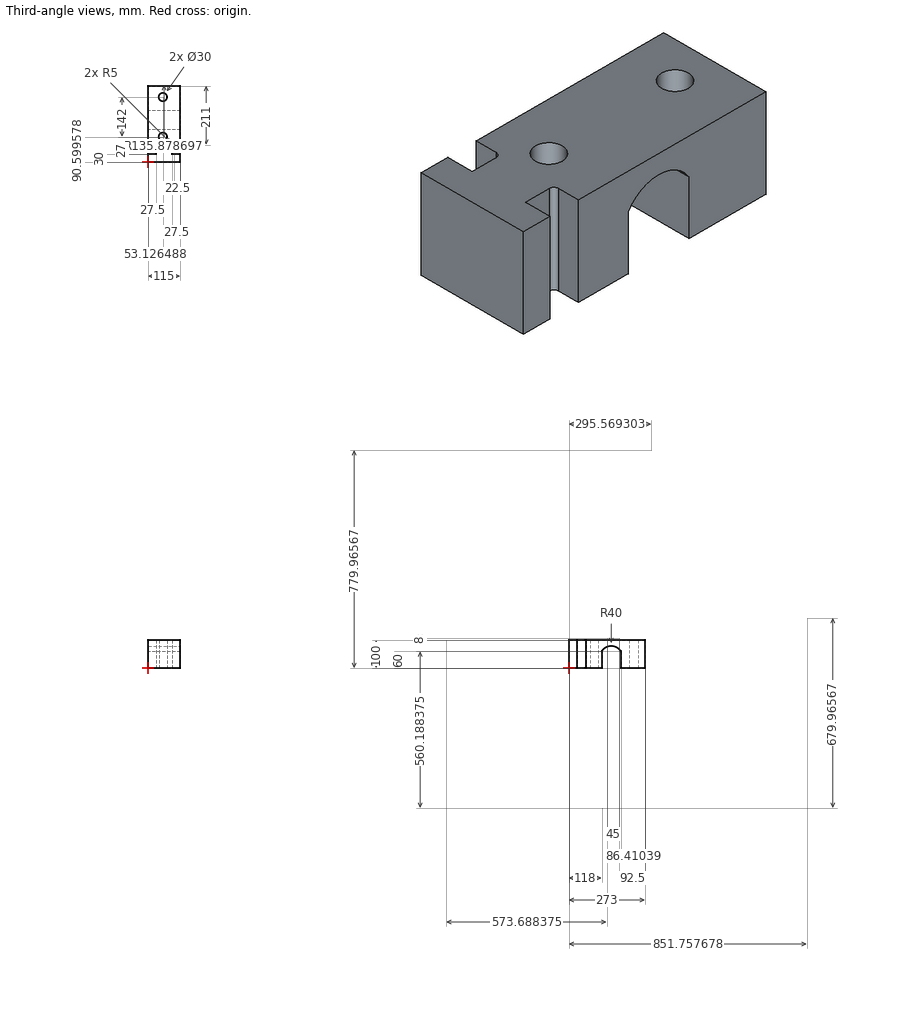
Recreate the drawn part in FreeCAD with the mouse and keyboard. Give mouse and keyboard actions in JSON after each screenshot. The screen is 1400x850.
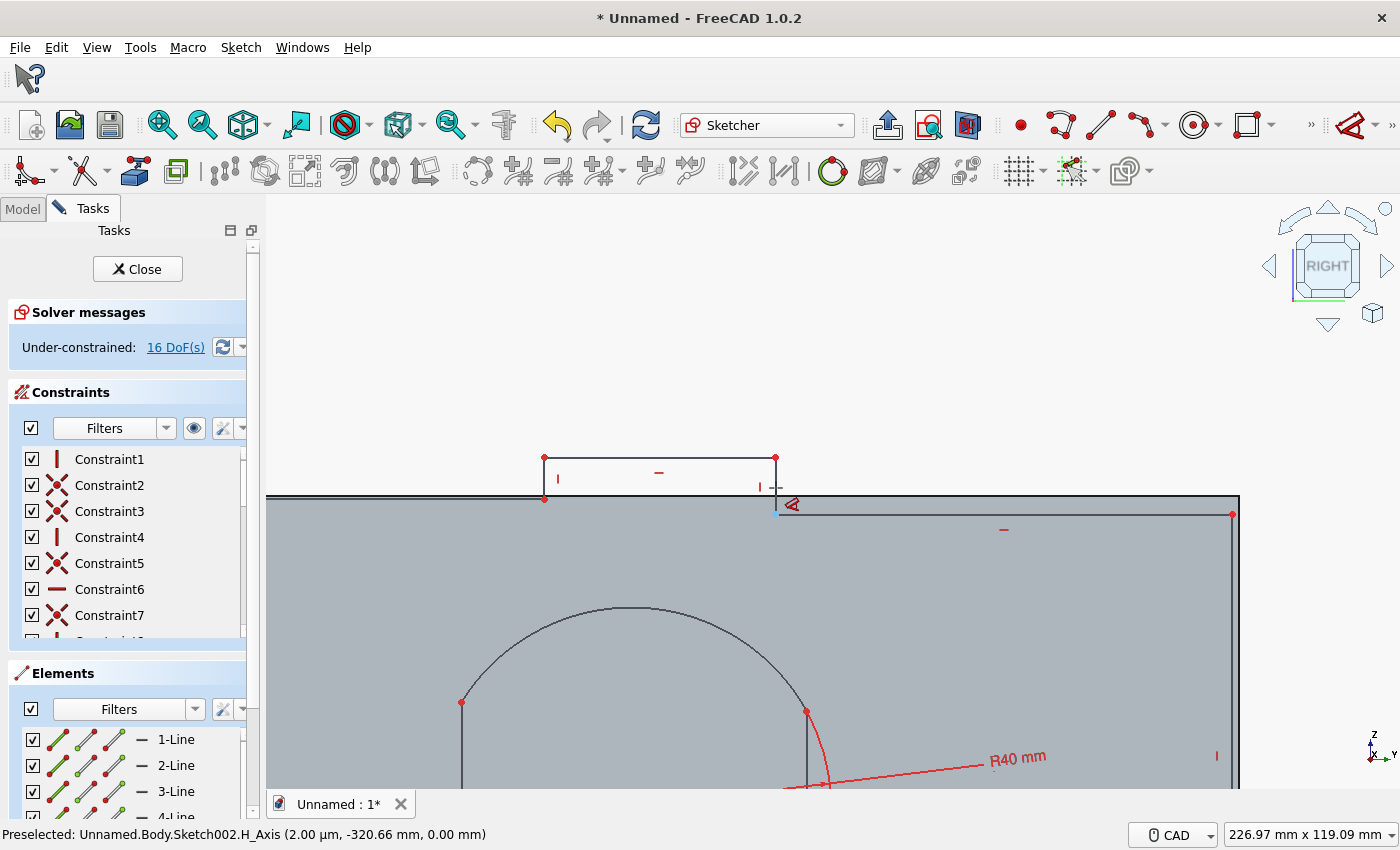
{"action": "left_click", "coordinate": [776, 486]}
{"action": "left_click", "coordinate": [742, 486]}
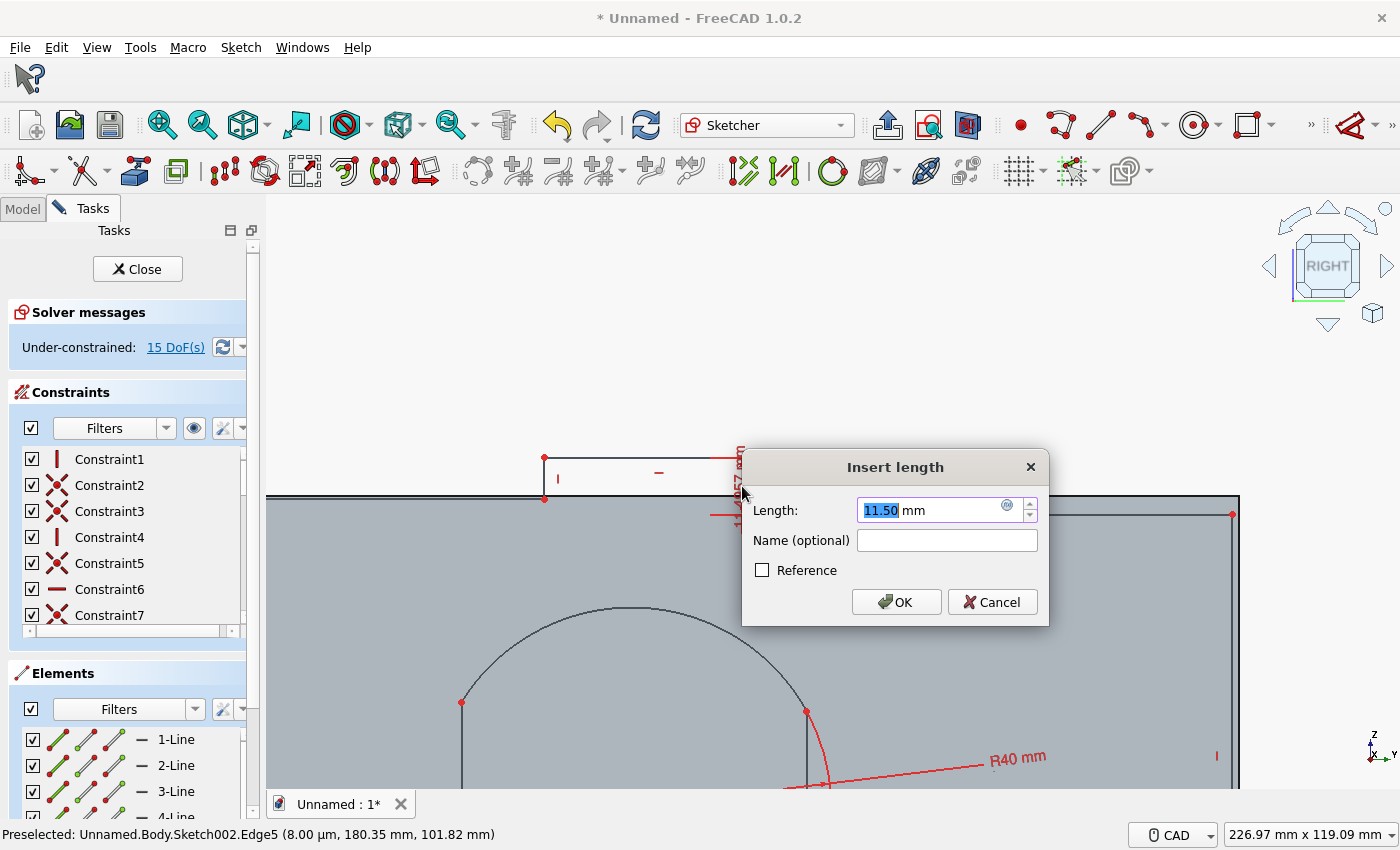
{"action": "type", "text": "8"}
{"action": "key", "text": "Return"}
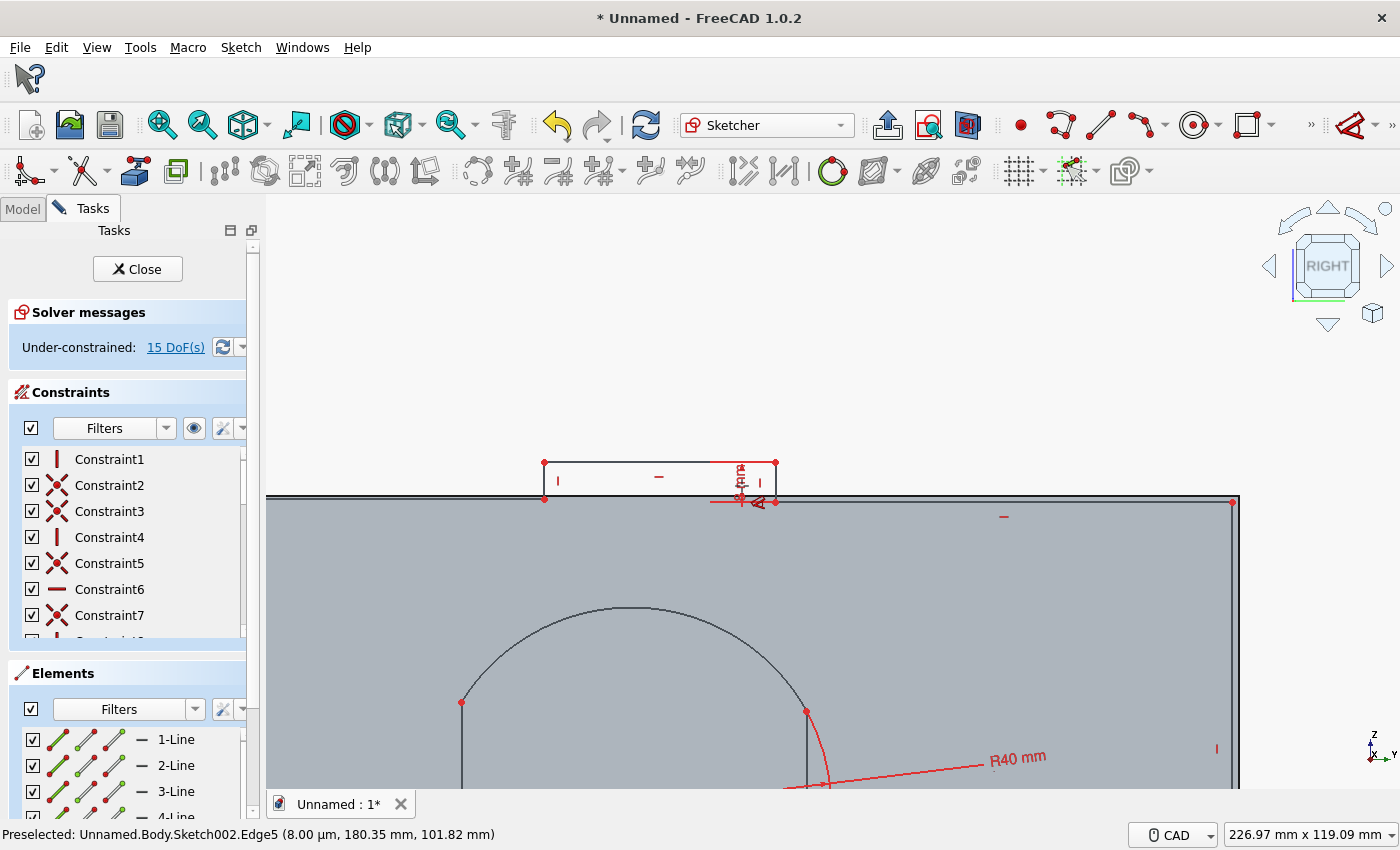
{"action": "left_click", "coordinate": [544, 473]}
{"action": "left_click", "coordinate": [510, 481]}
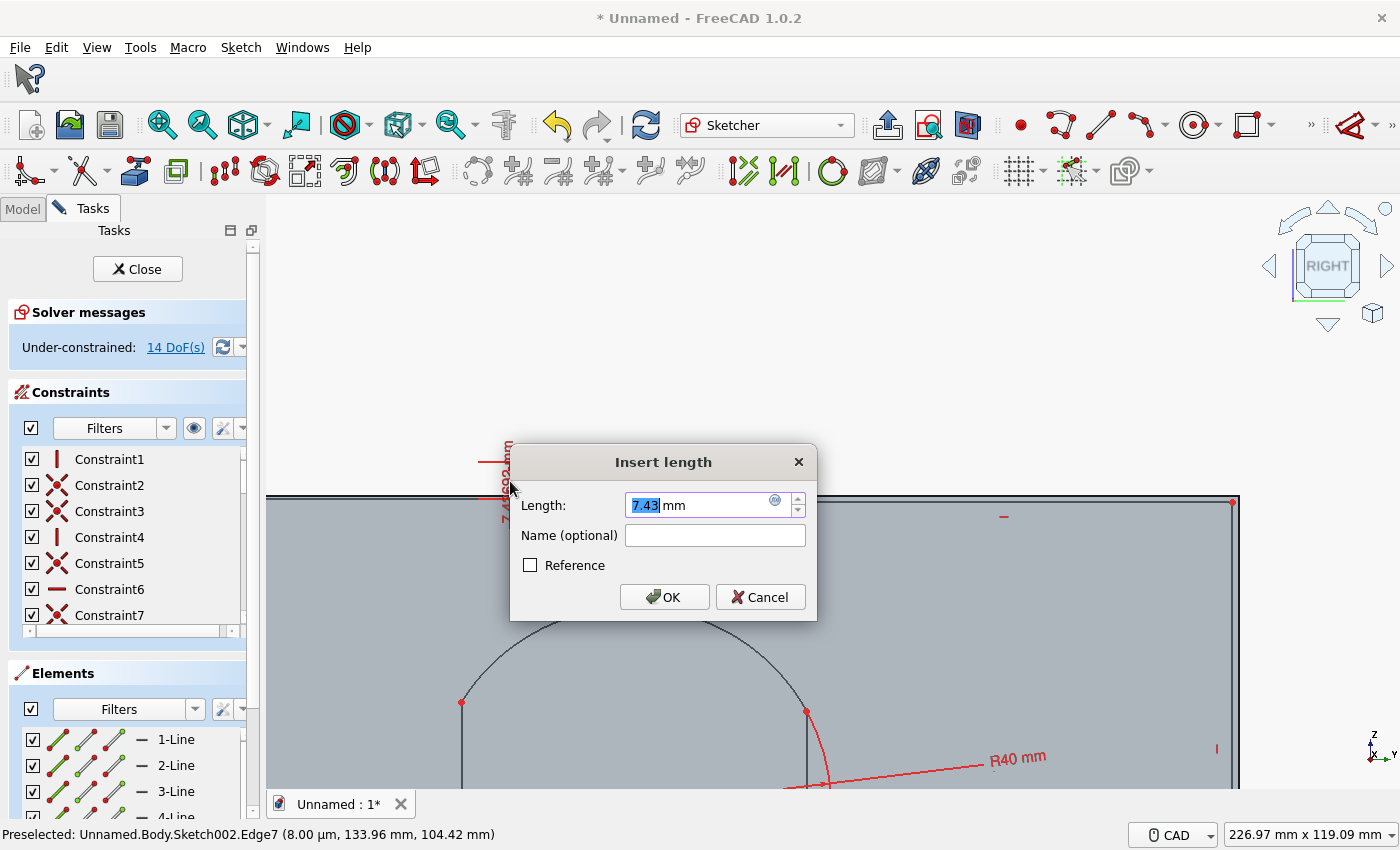
{"action": "type", "text": "8"}
{"action": "key", "text": "Return"}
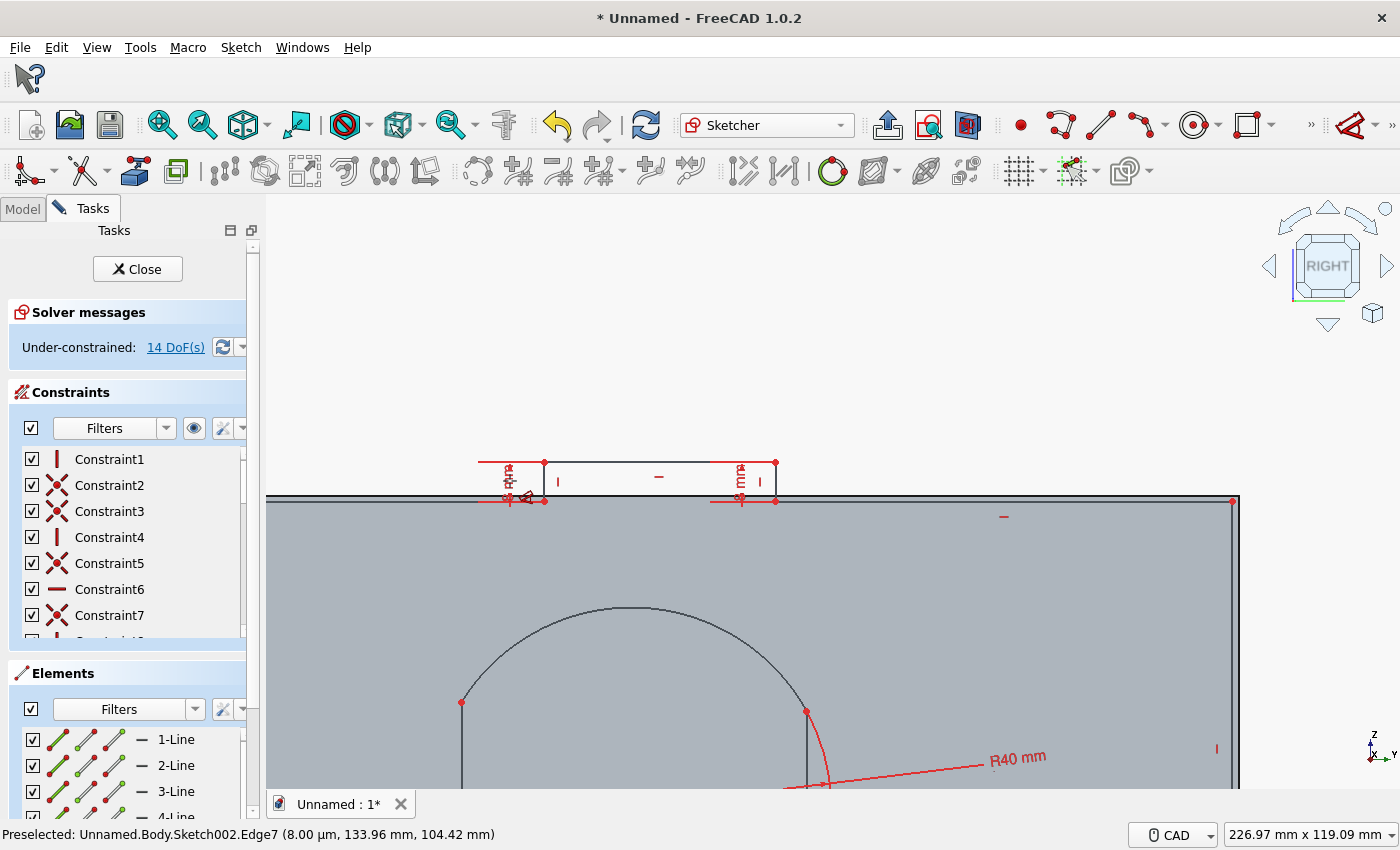
{"action": "scroll", "coordinate": [755, 504], "scroll_direction": "down", "scroll_amount": 14}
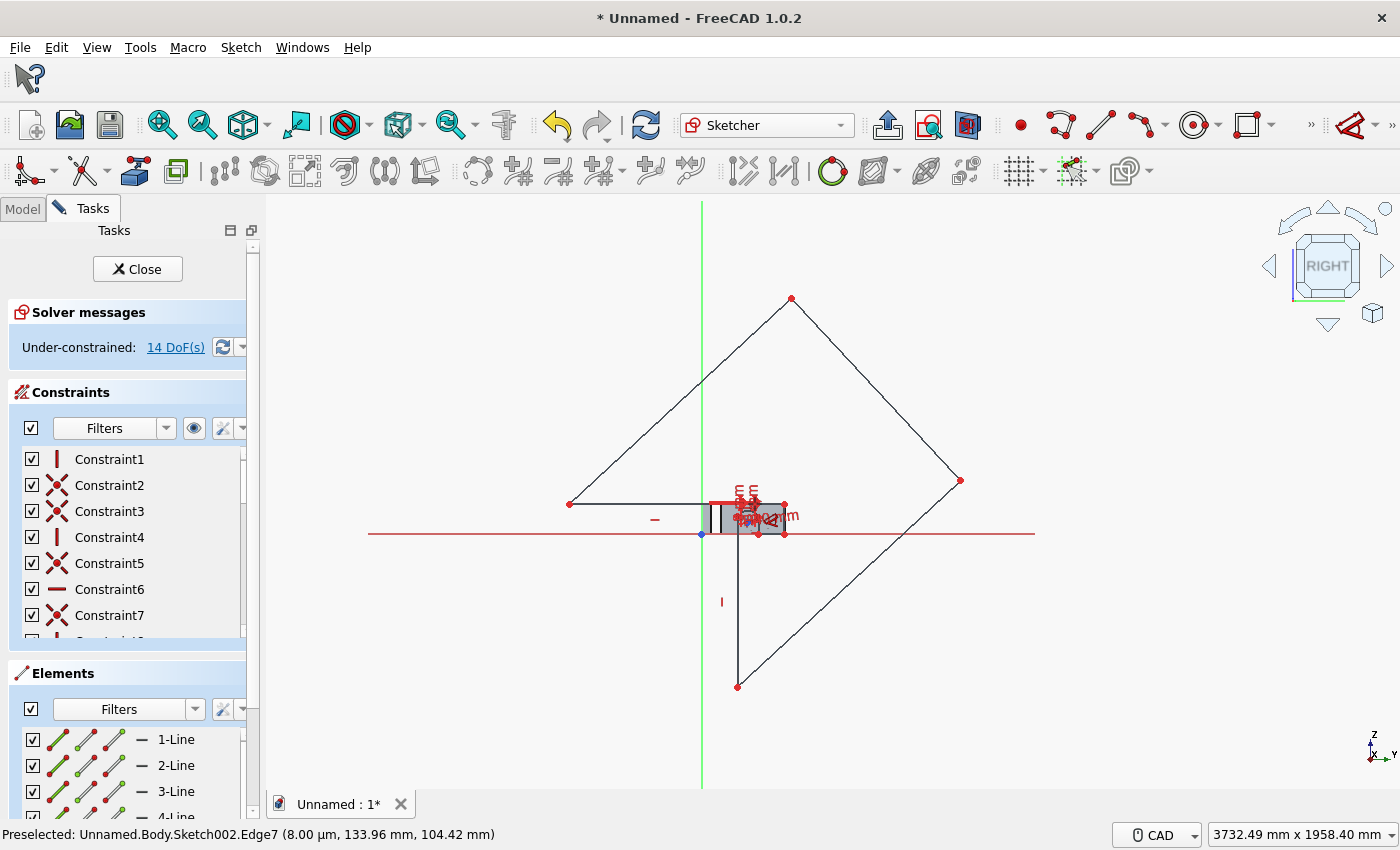
{"action": "scroll", "coordinate": [759, 522], "scroll_direction": "up", "scroll_amount": 5}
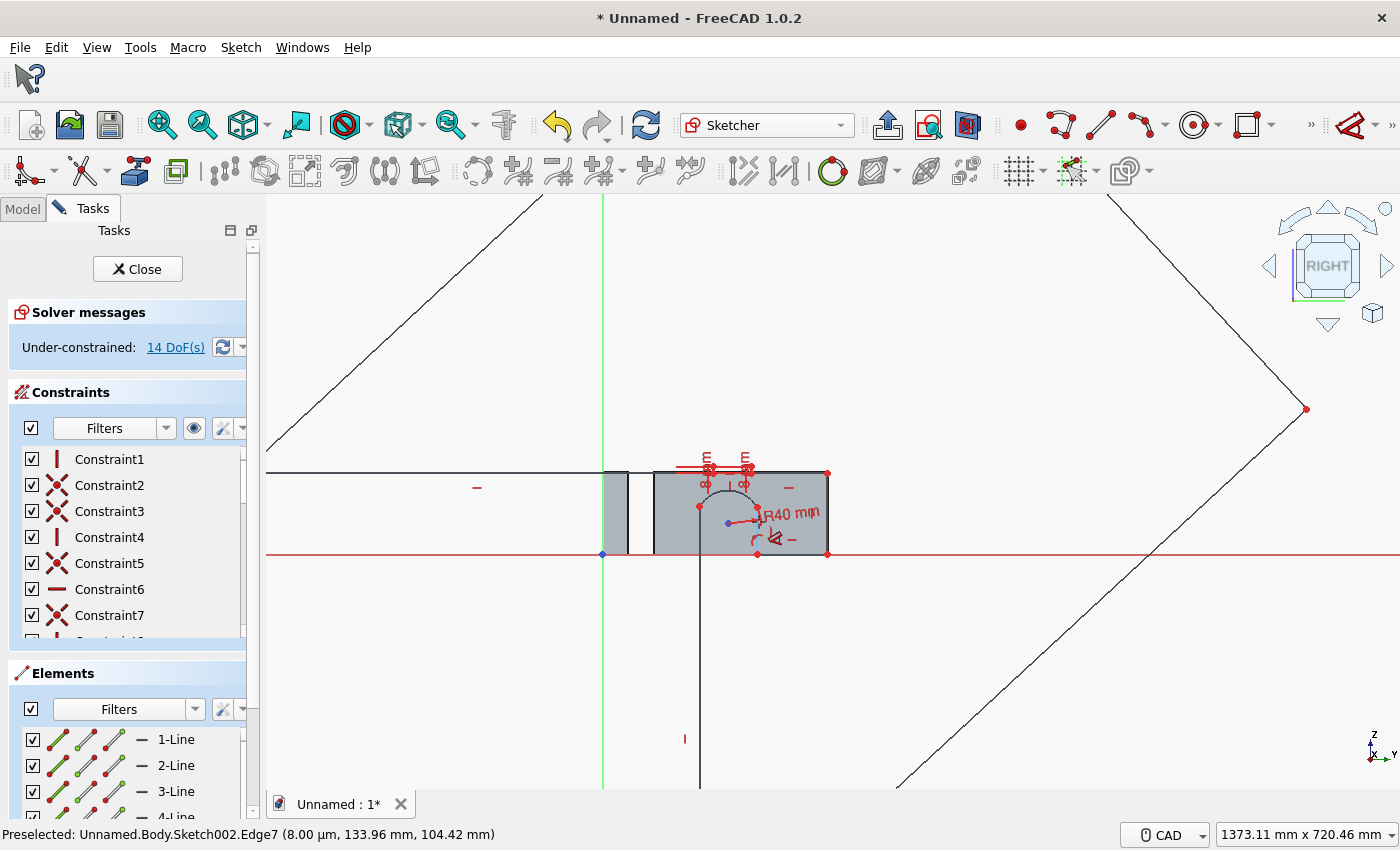
{"action": "left_click", "coordinate": [757, 522]}
{"action": "left_click", "coordinate": [675, 531]}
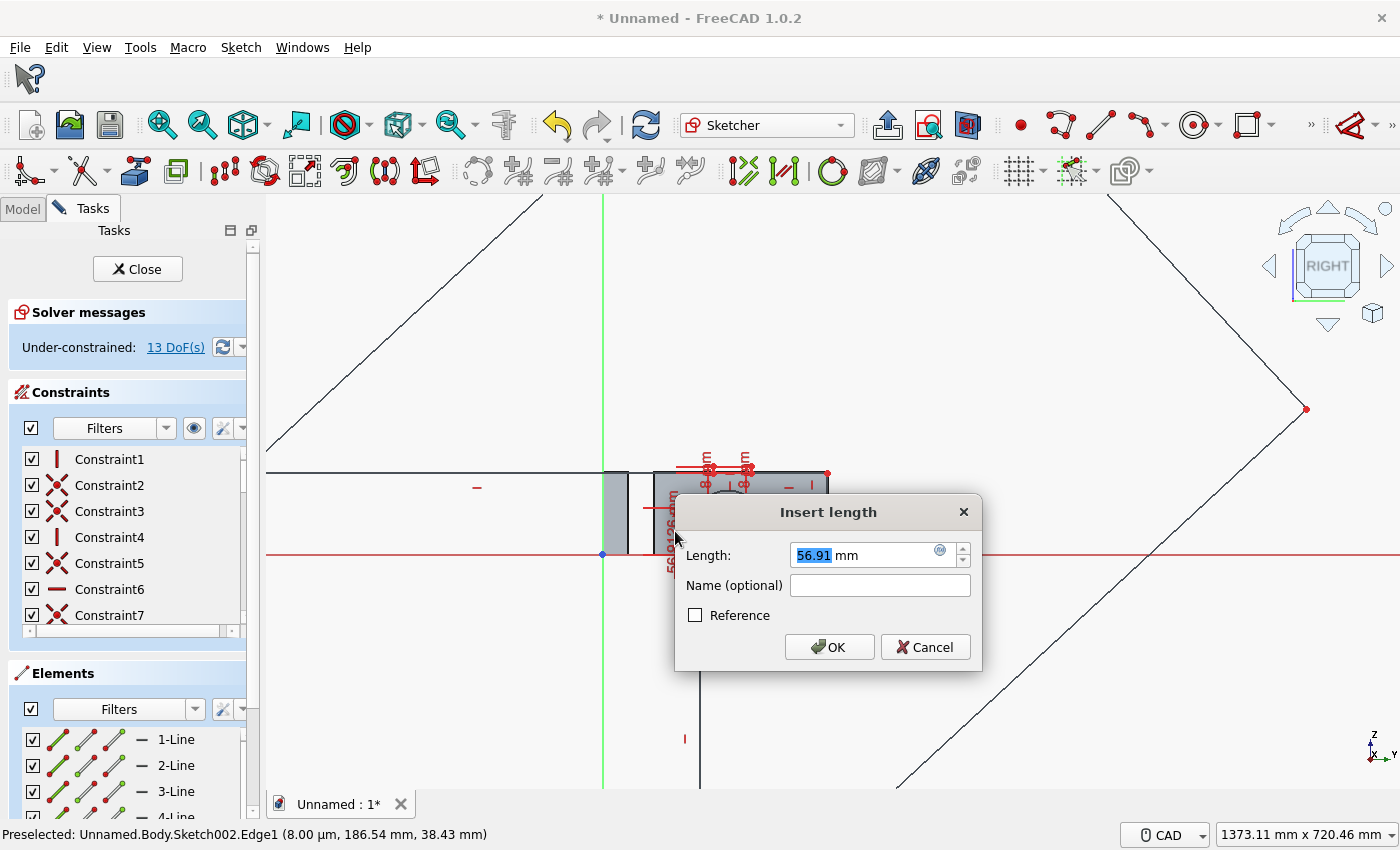
{"action": "type", "text": "60"}
{"action": "key", "text": "Return"}